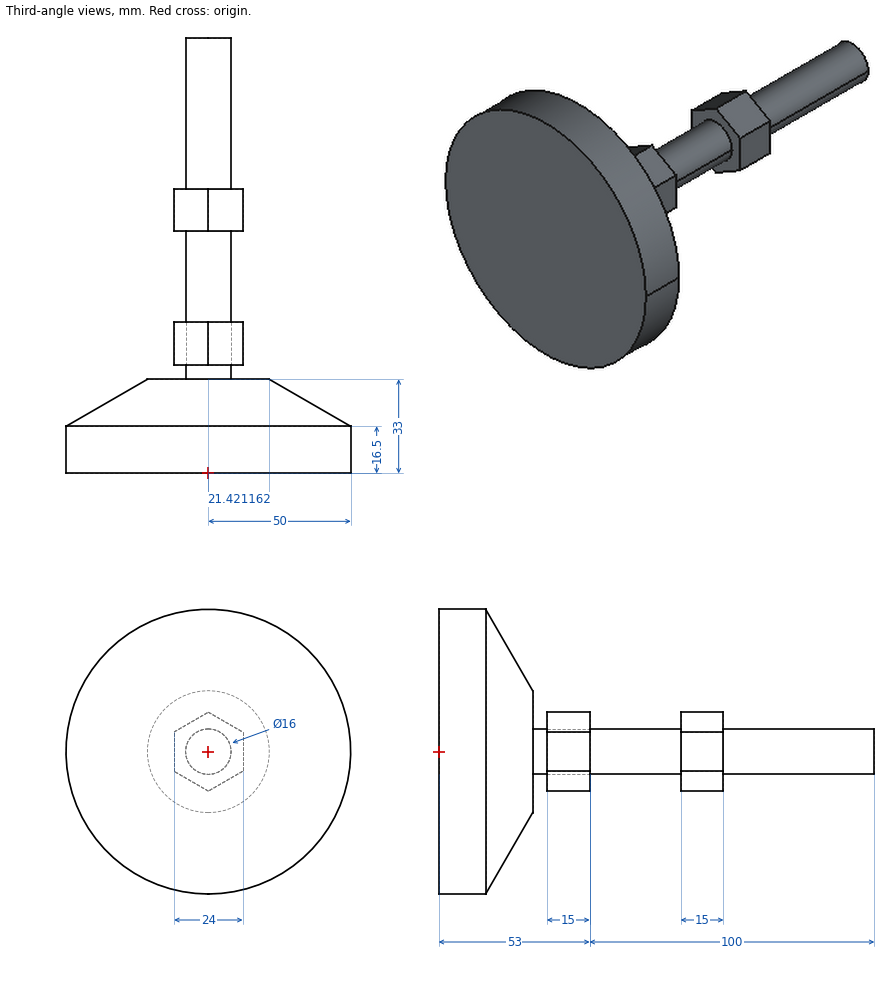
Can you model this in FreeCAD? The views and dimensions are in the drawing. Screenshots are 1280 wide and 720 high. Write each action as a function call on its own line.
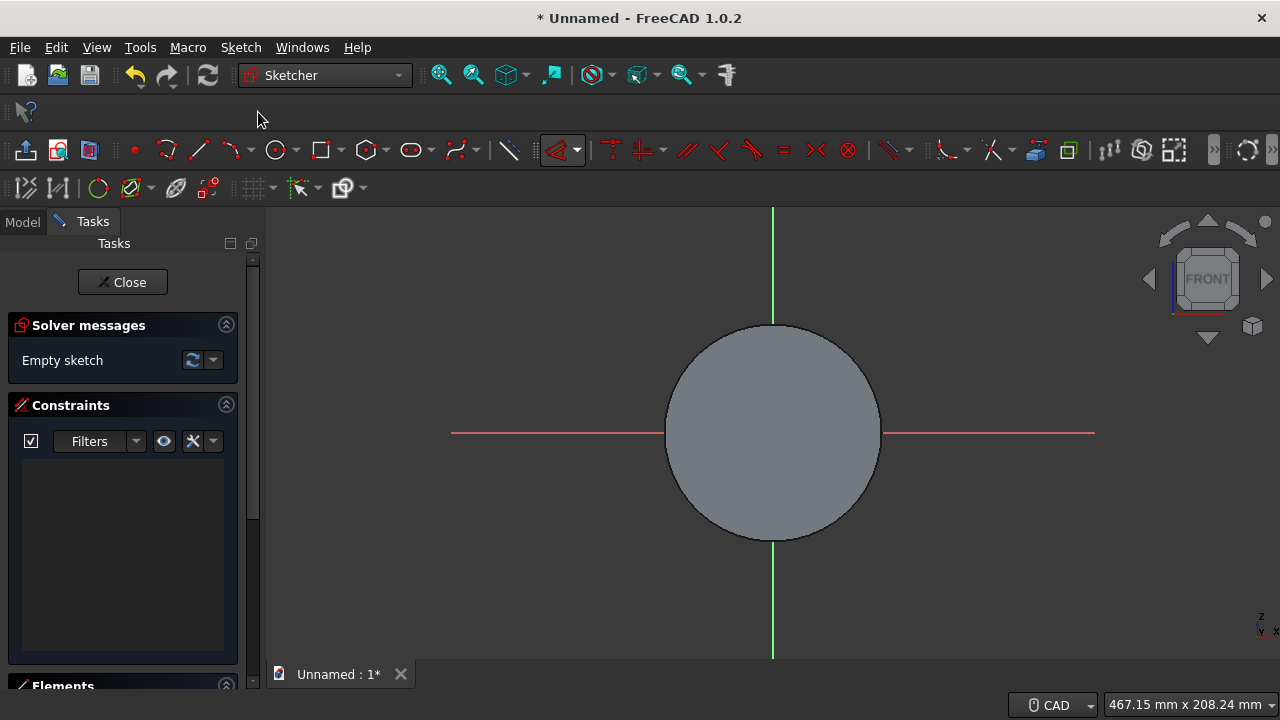
scroll(790, 433, up, 8)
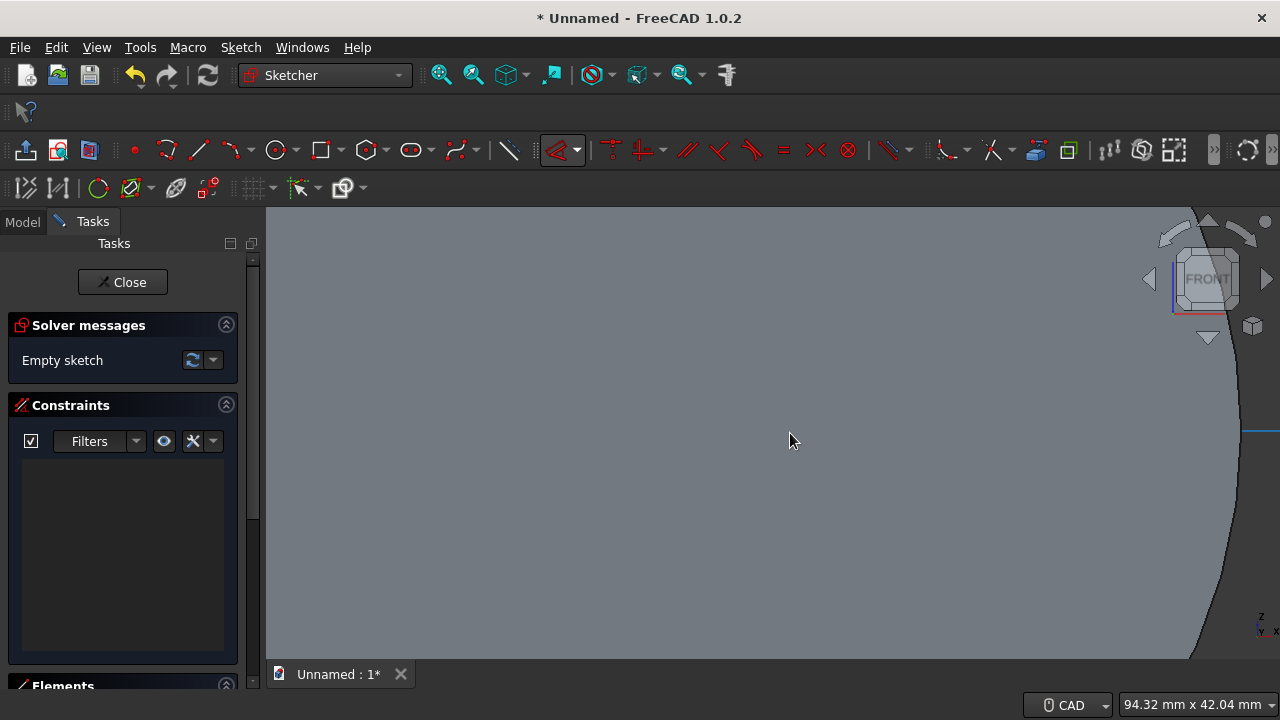
click(366, 150)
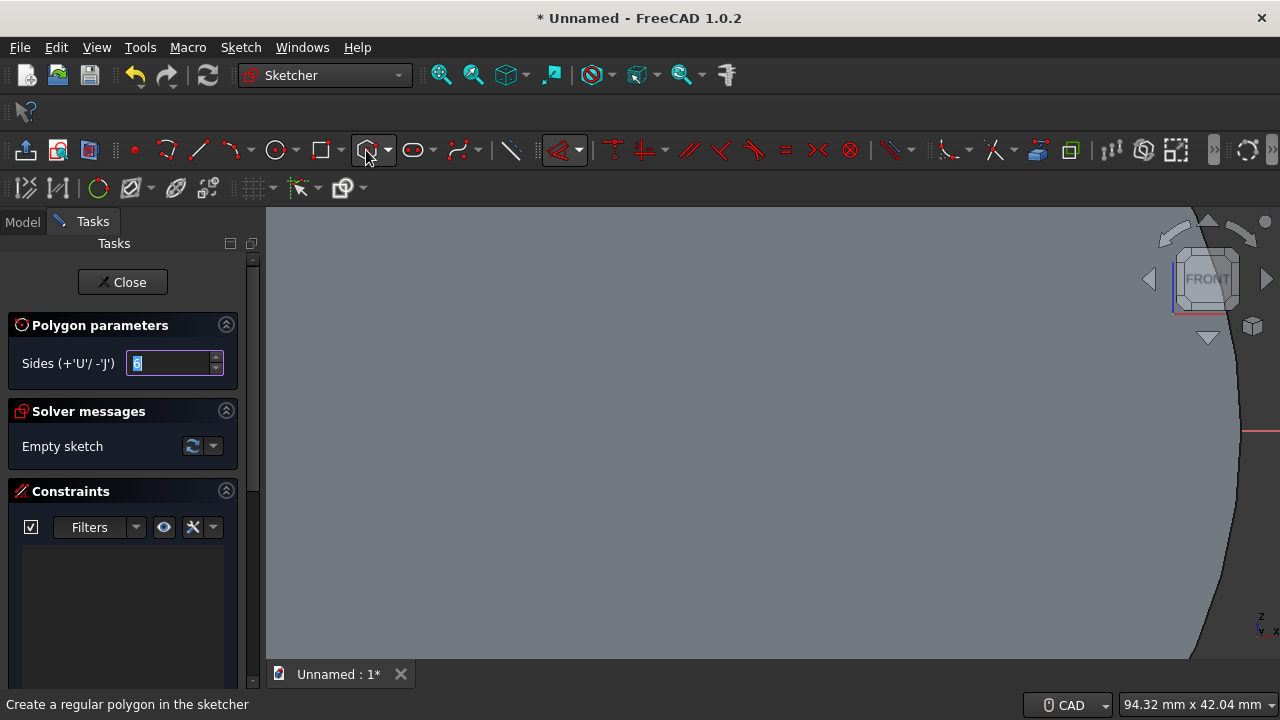
click(704, 431)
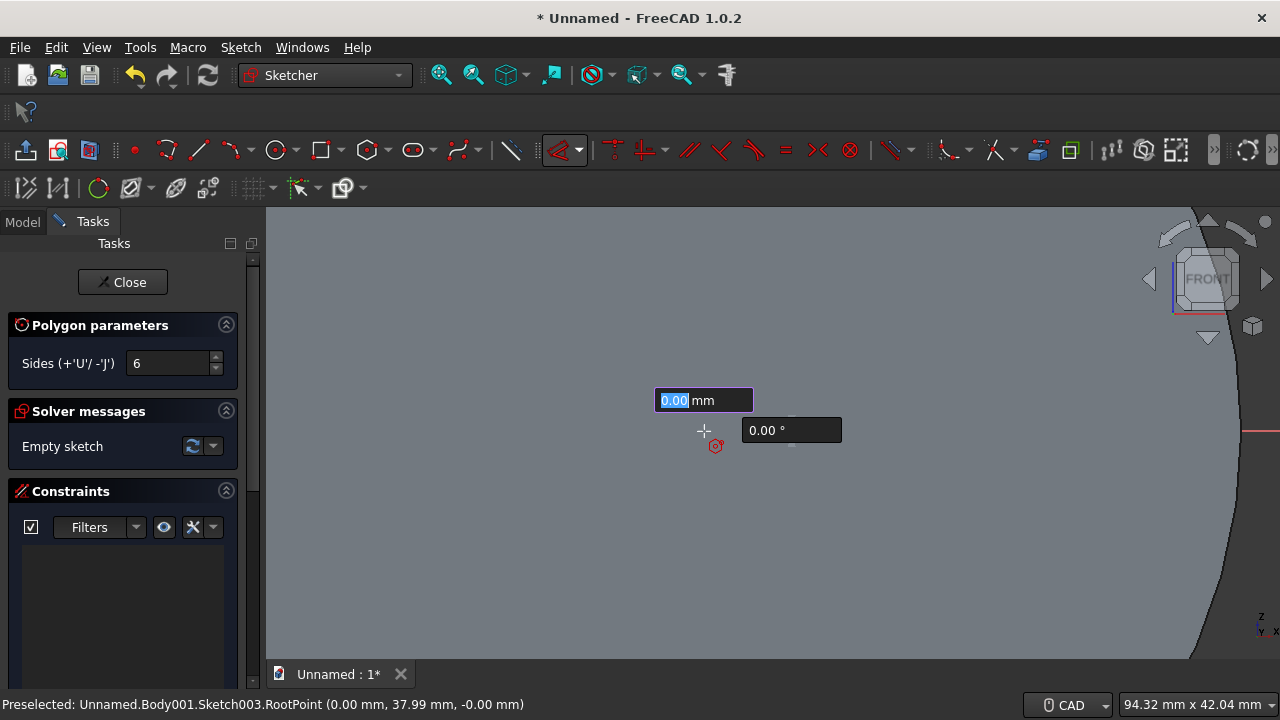
click(704, 580)
key(Escape)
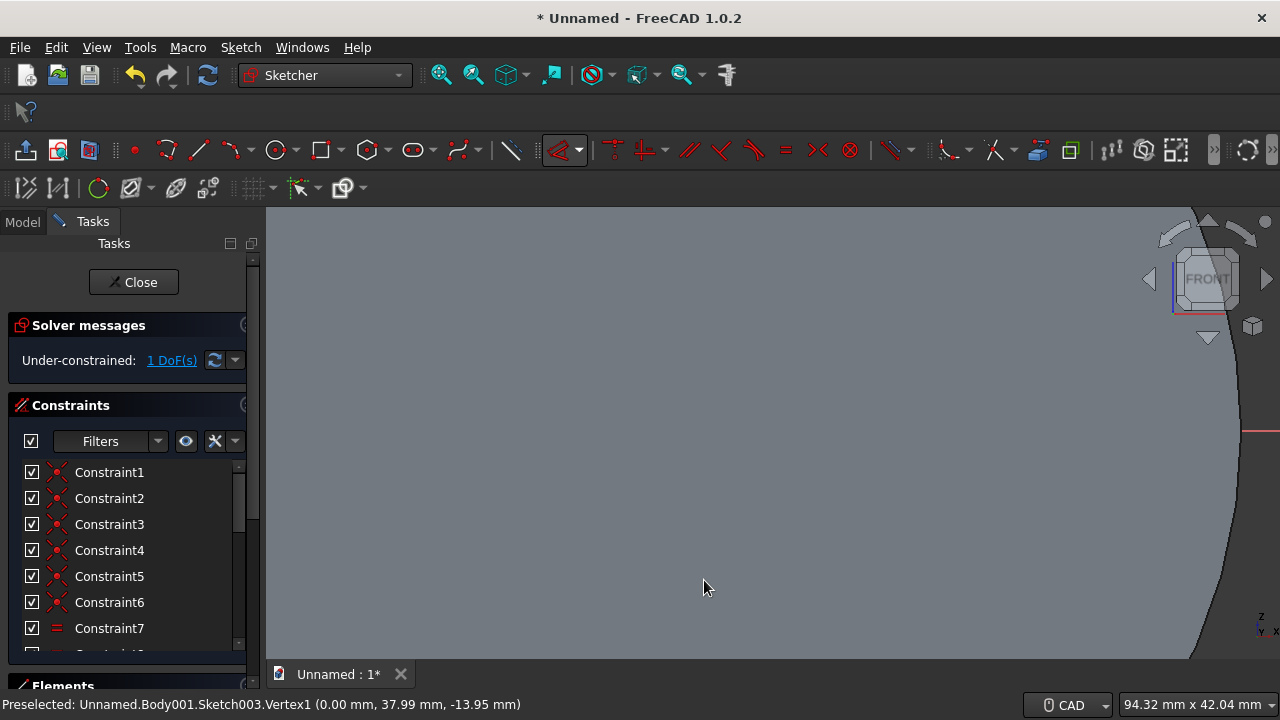
click(574, 356)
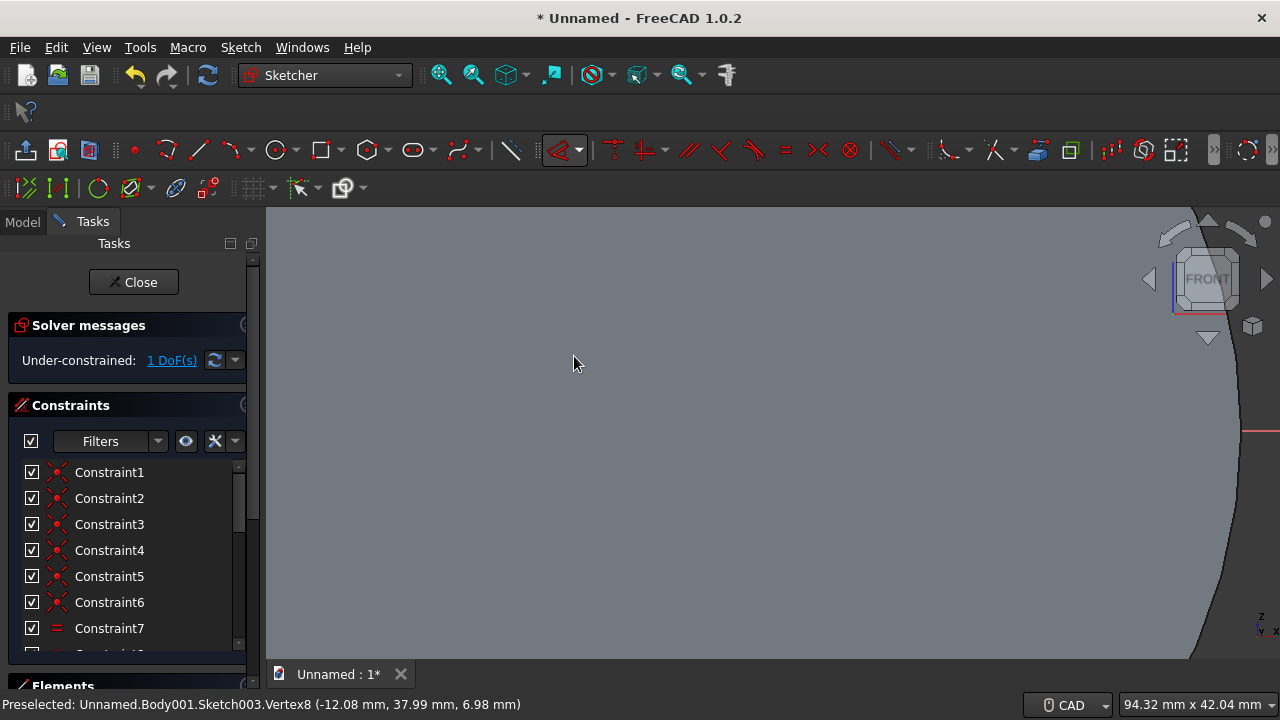
click(834, 506)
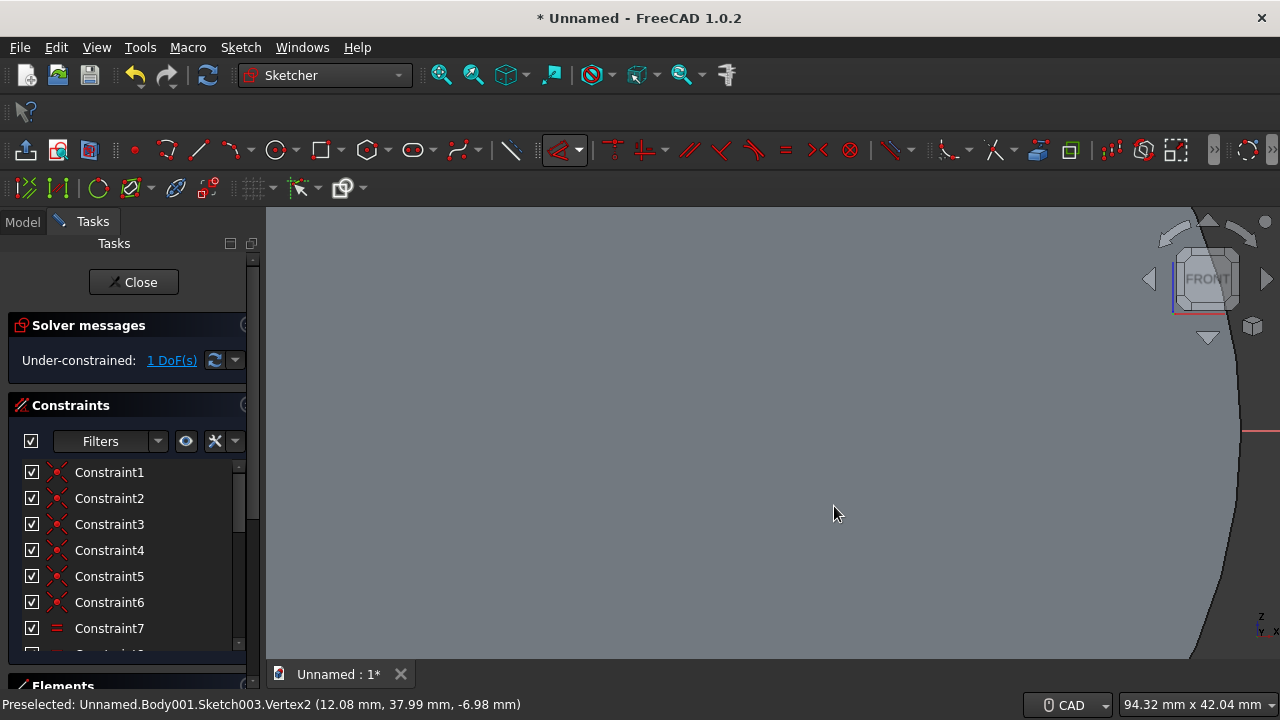
key(l)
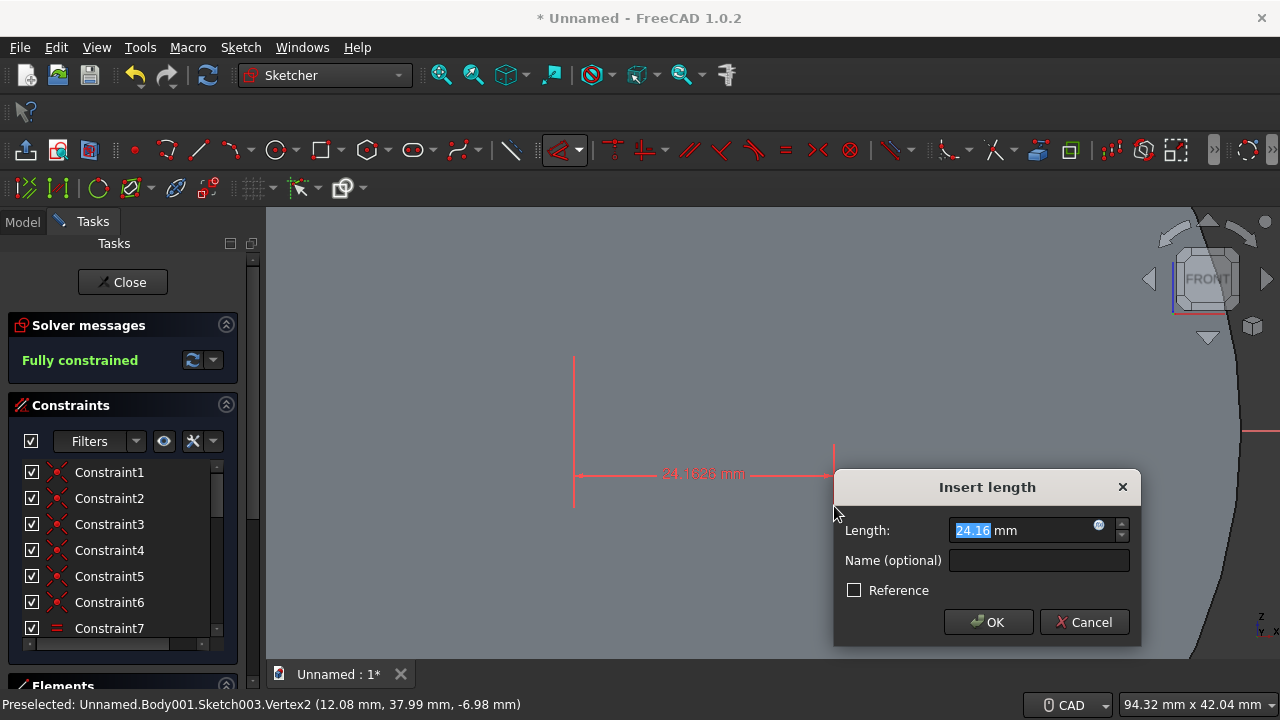
text(24)
key(Return)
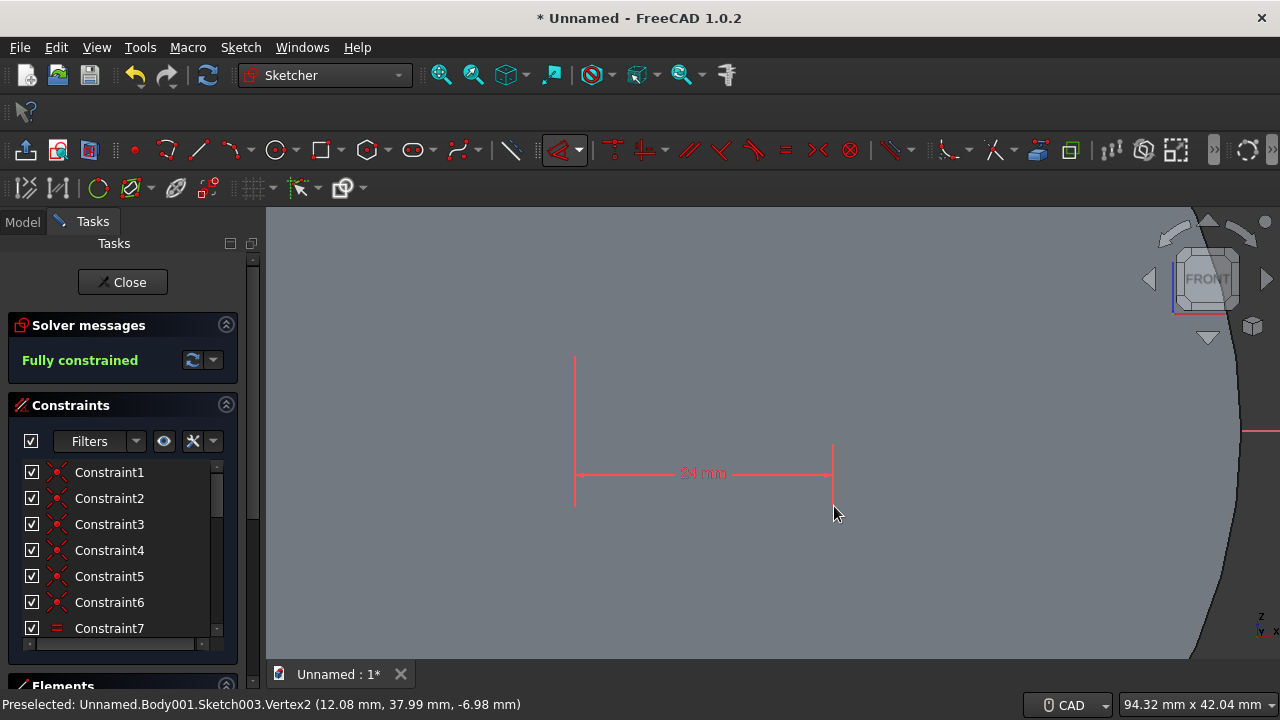
click(123, 282)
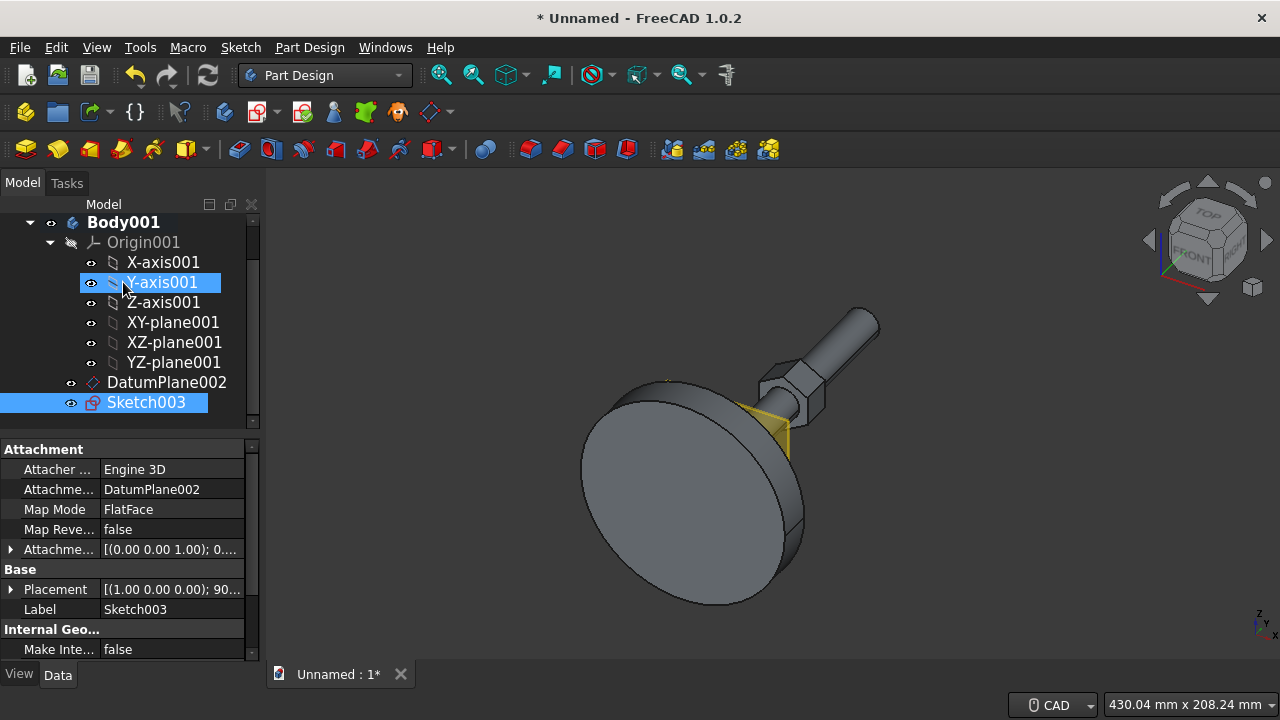
click(26, 150)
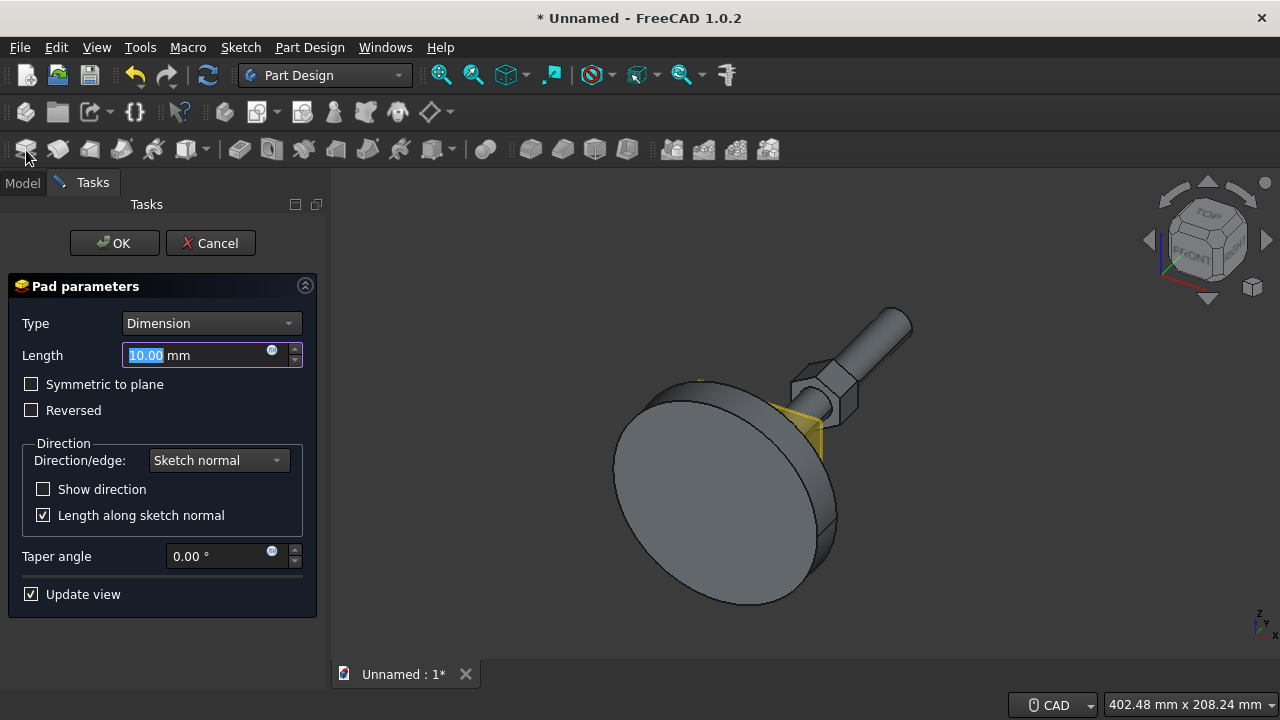
text(15)
key(Tab)